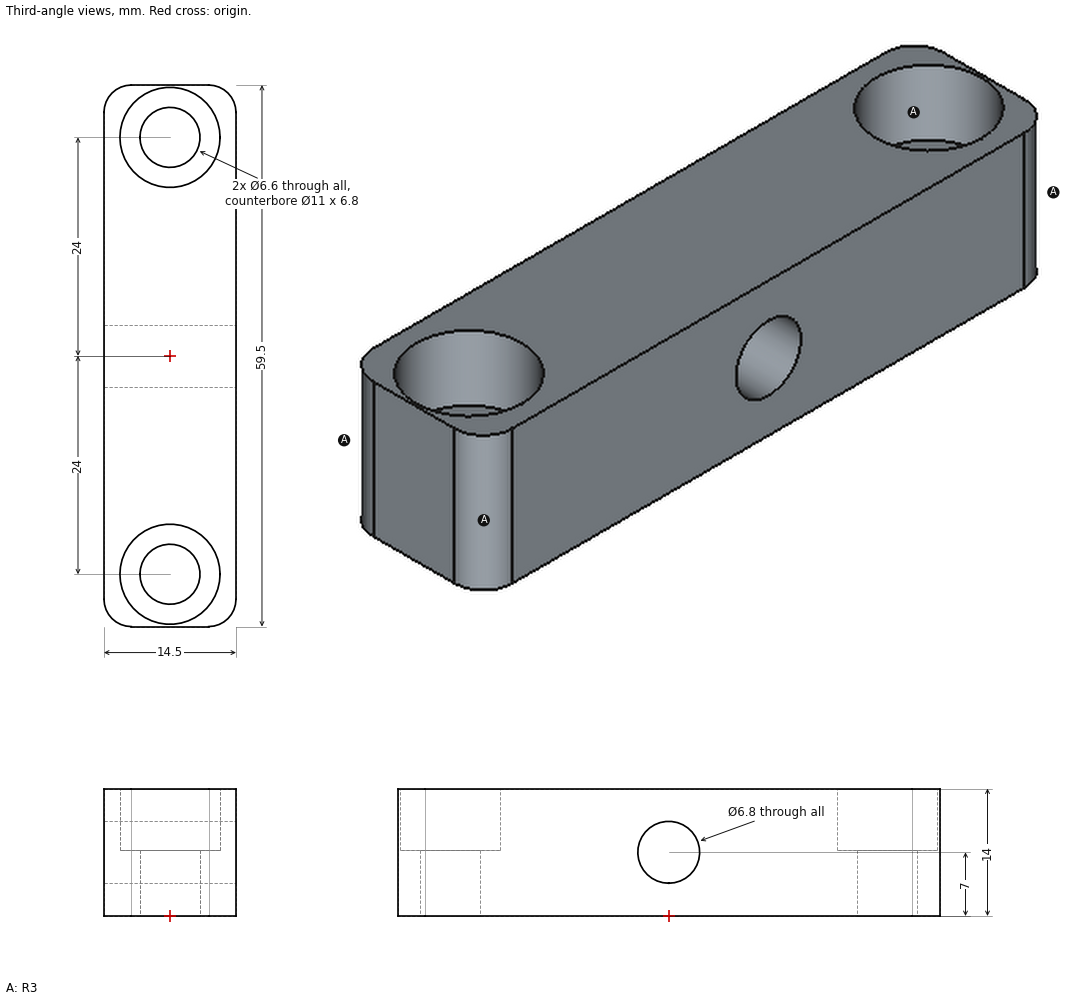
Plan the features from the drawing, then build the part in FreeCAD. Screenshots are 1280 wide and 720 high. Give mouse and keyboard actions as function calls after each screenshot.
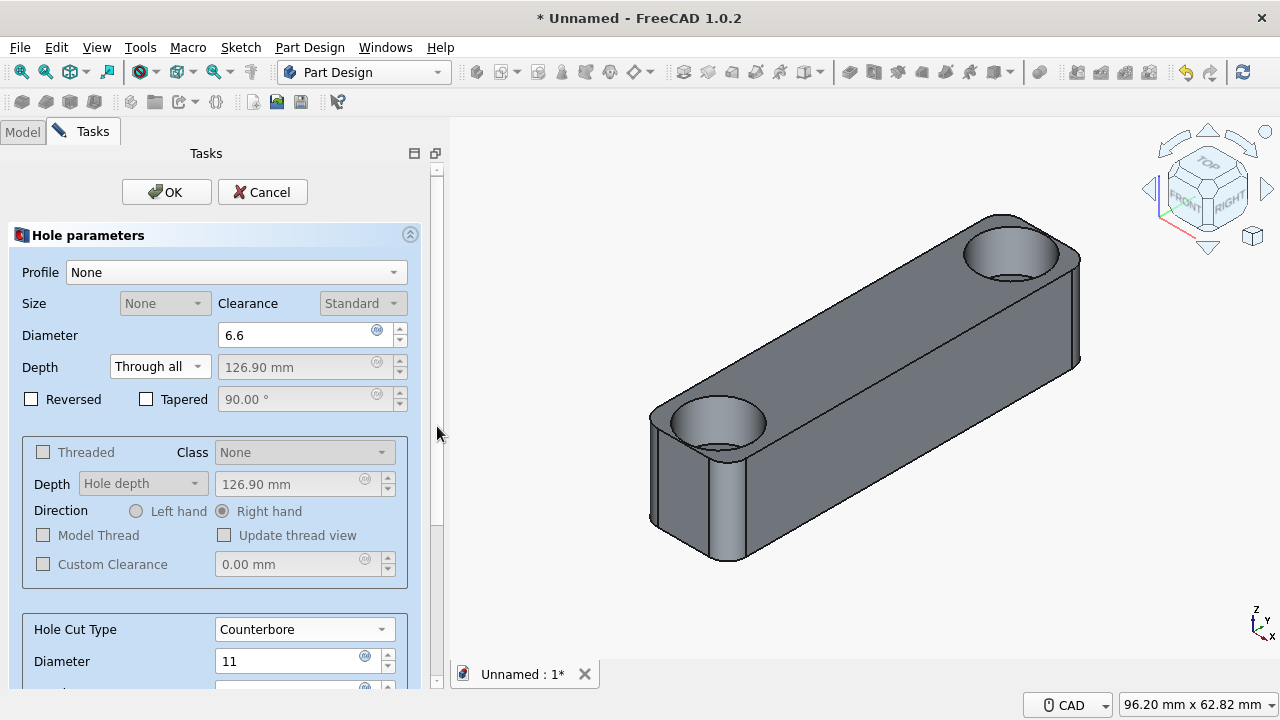
click(167, 192)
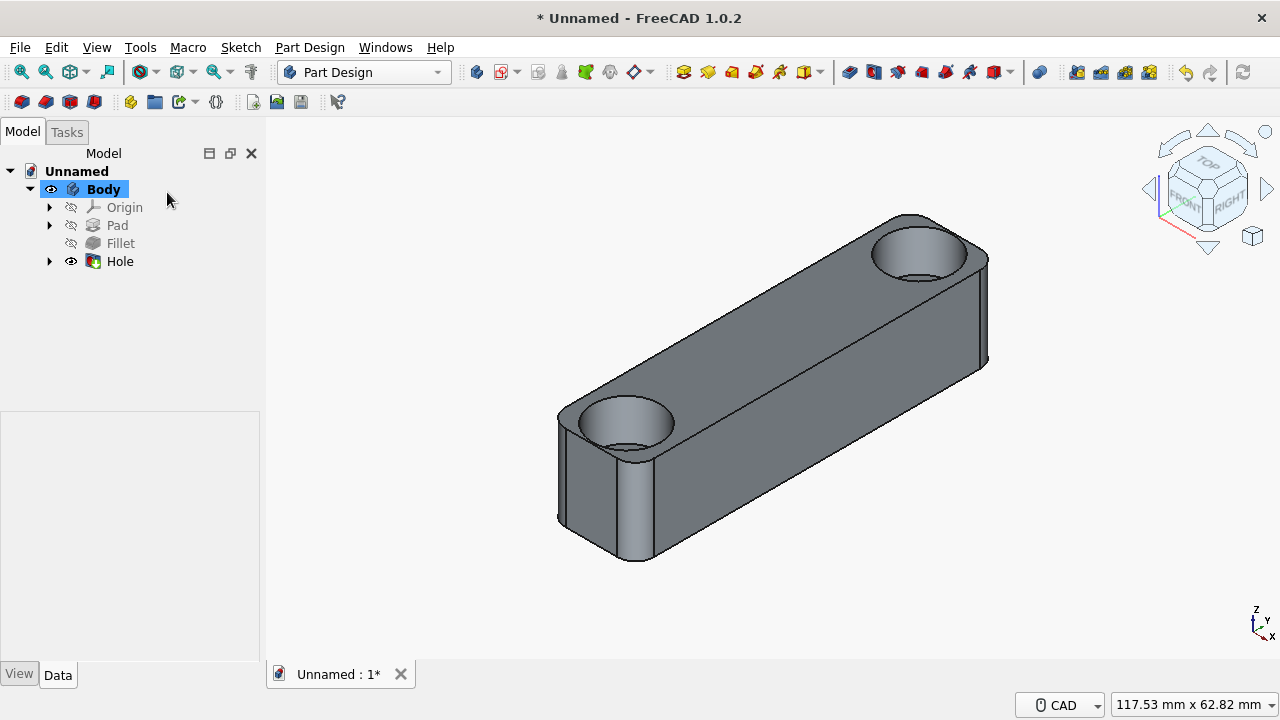
key(6)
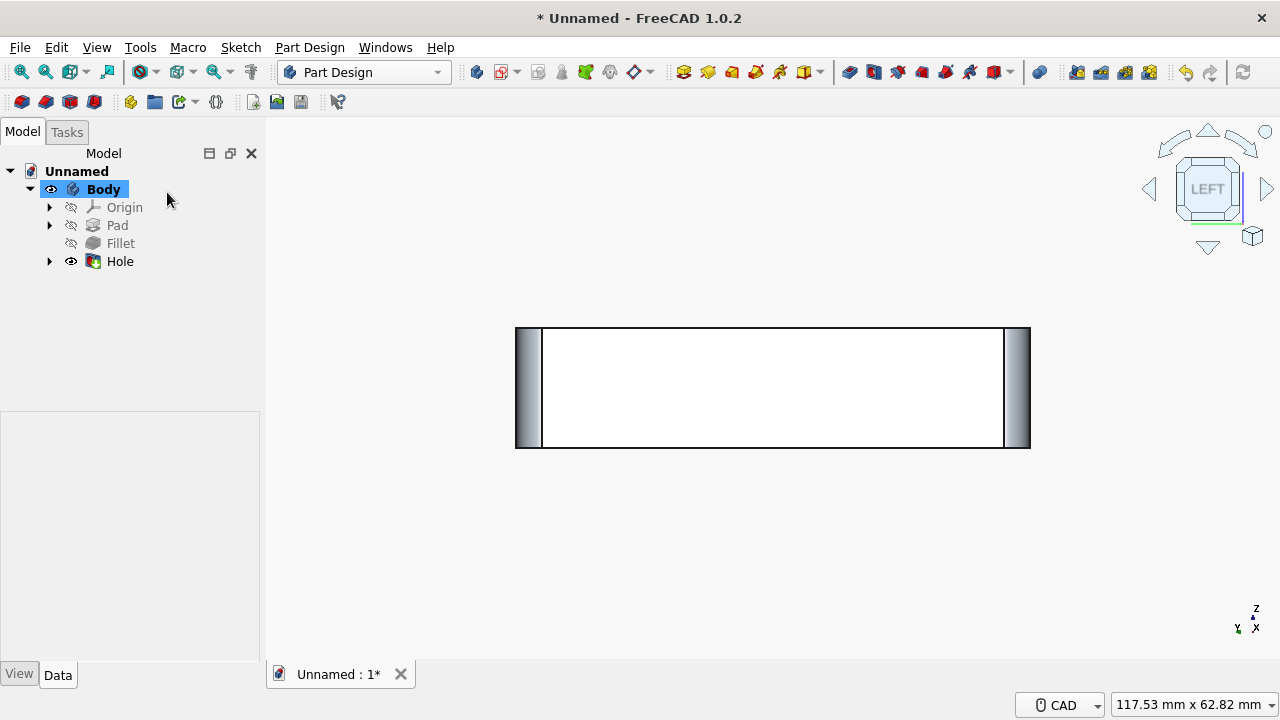
click(641, 387)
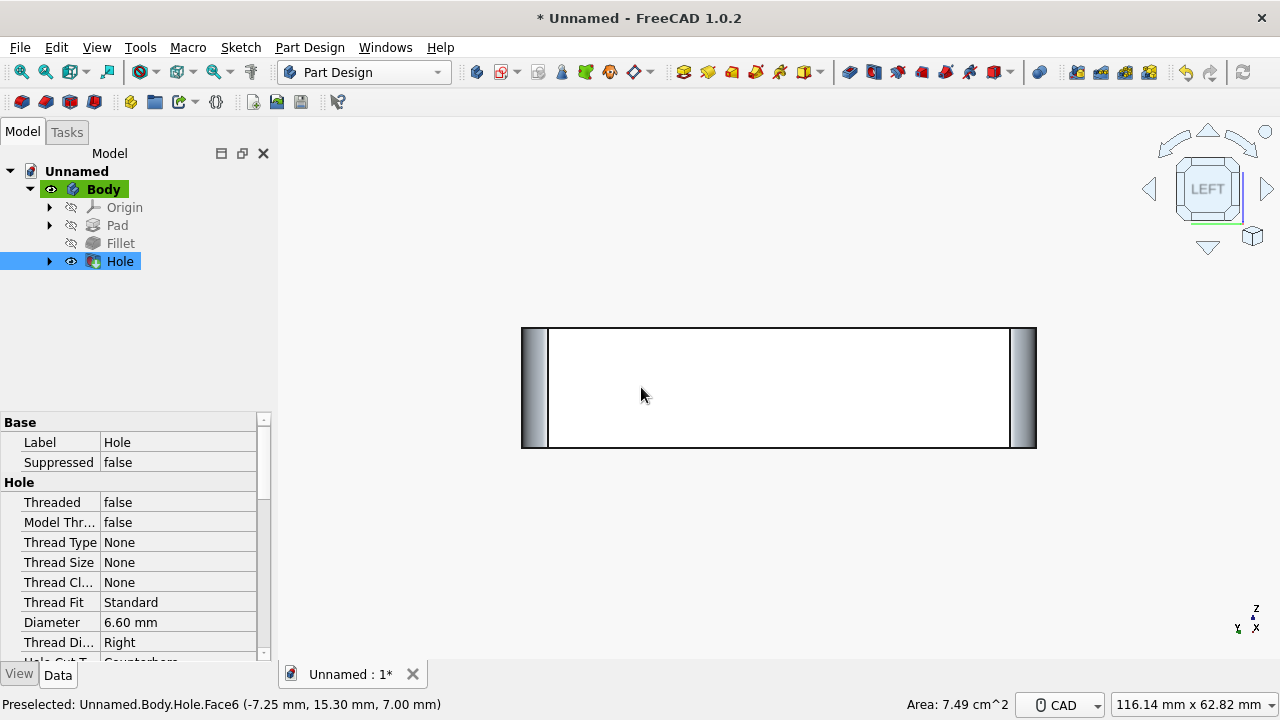
click(502, 72)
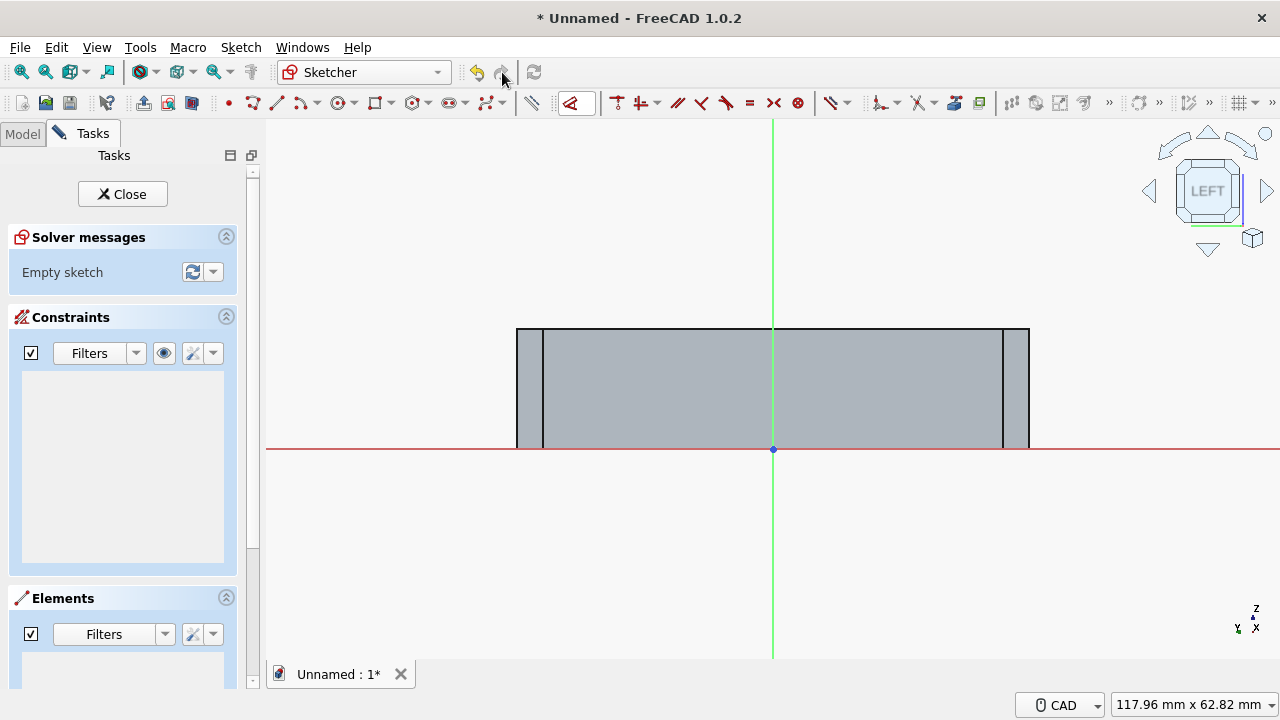
scroll(795, 410, up, 7)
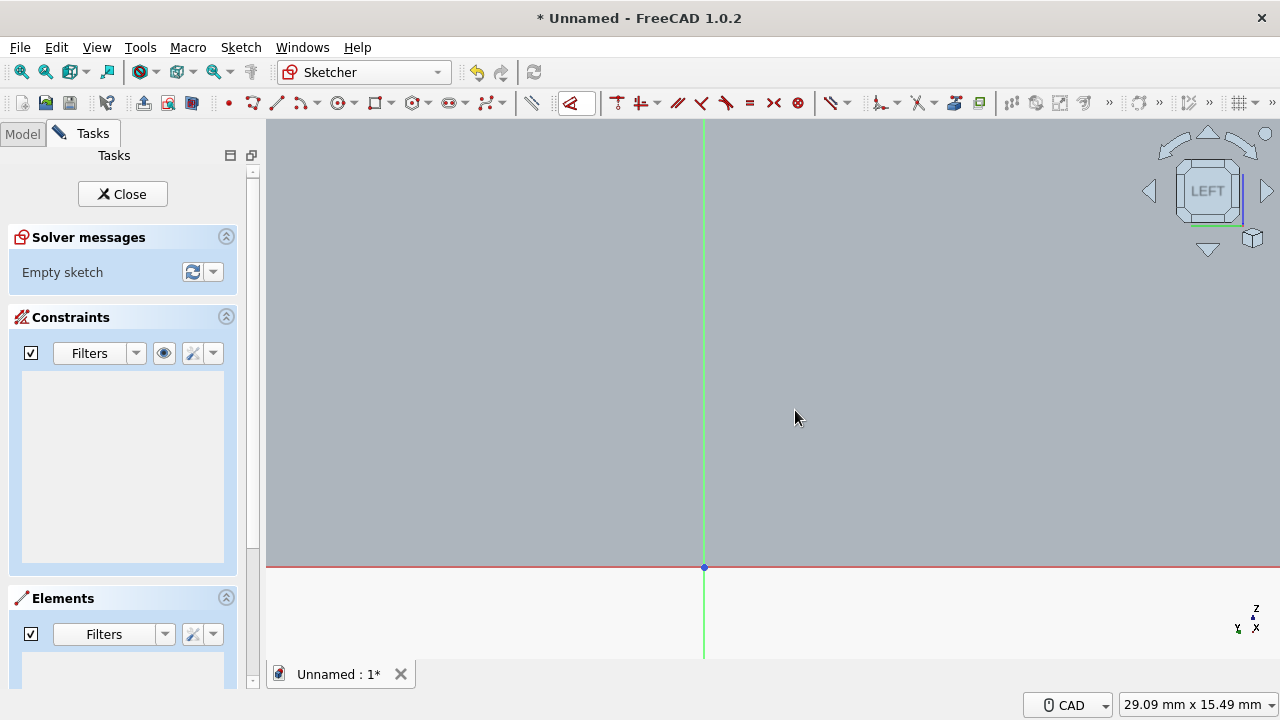
key(g)
key(c)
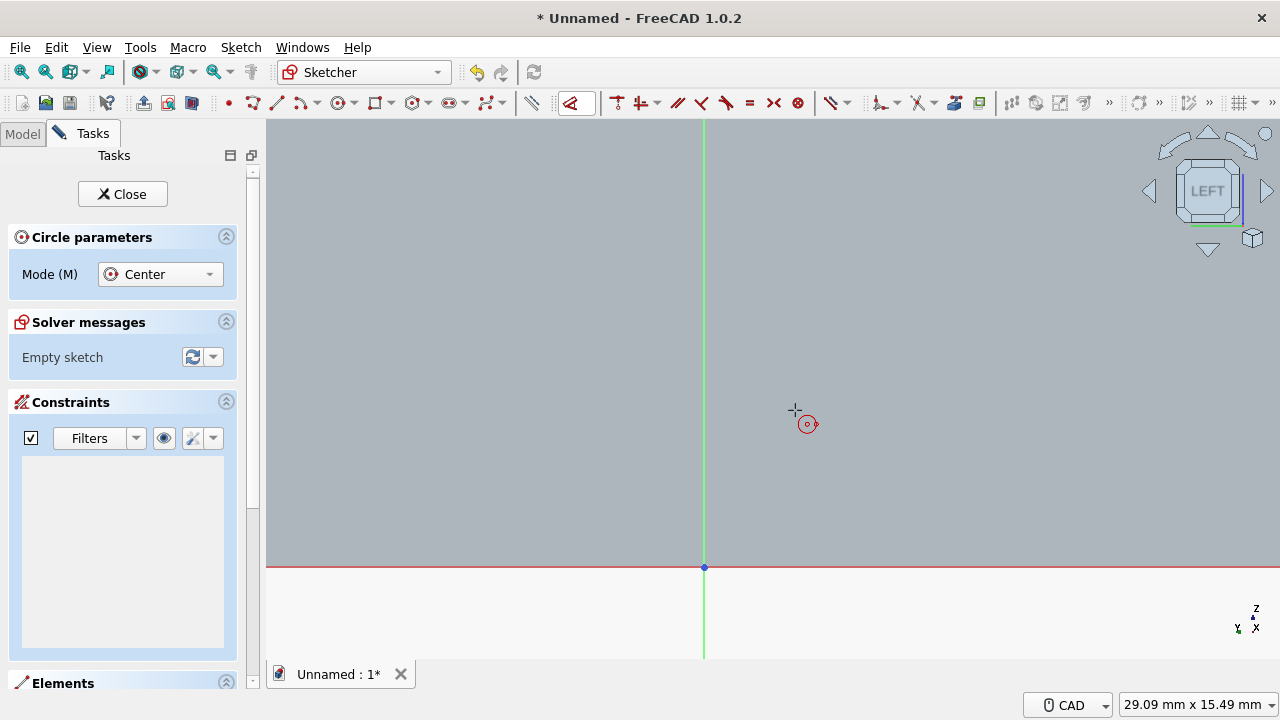
click(704, 323)
move(788, 239)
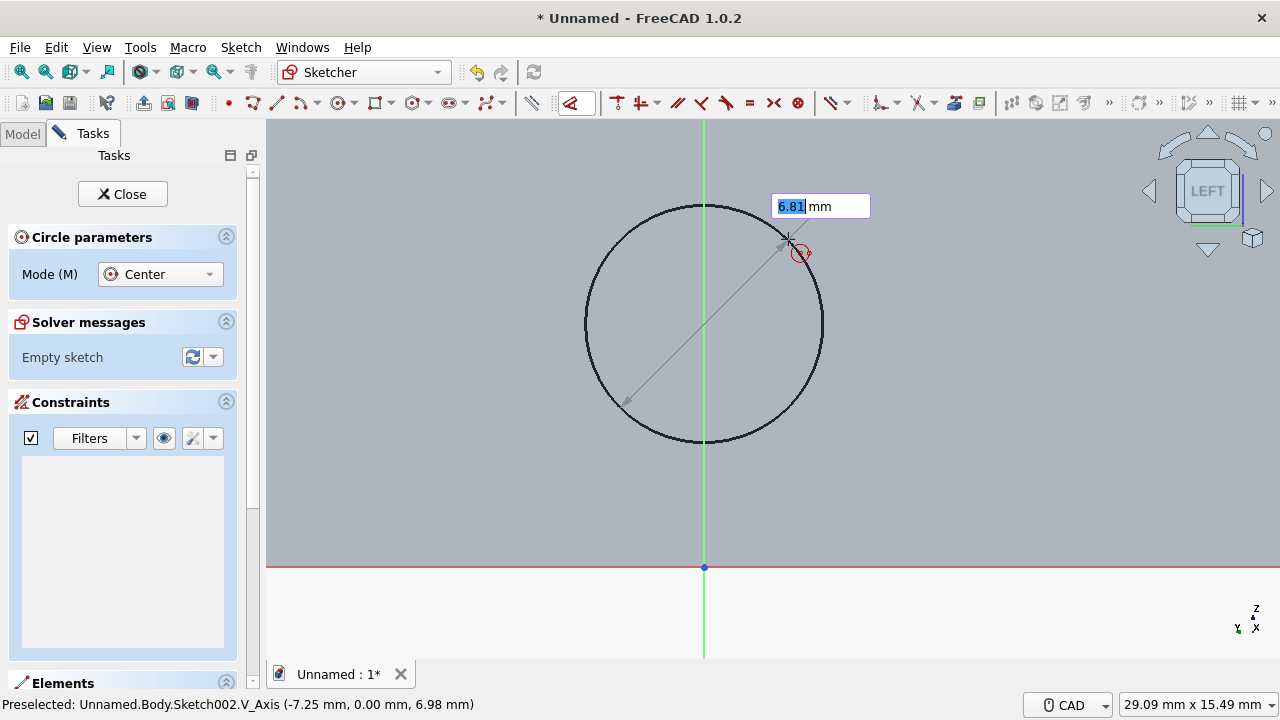
text(6.8)
key(Return)
key(Escape)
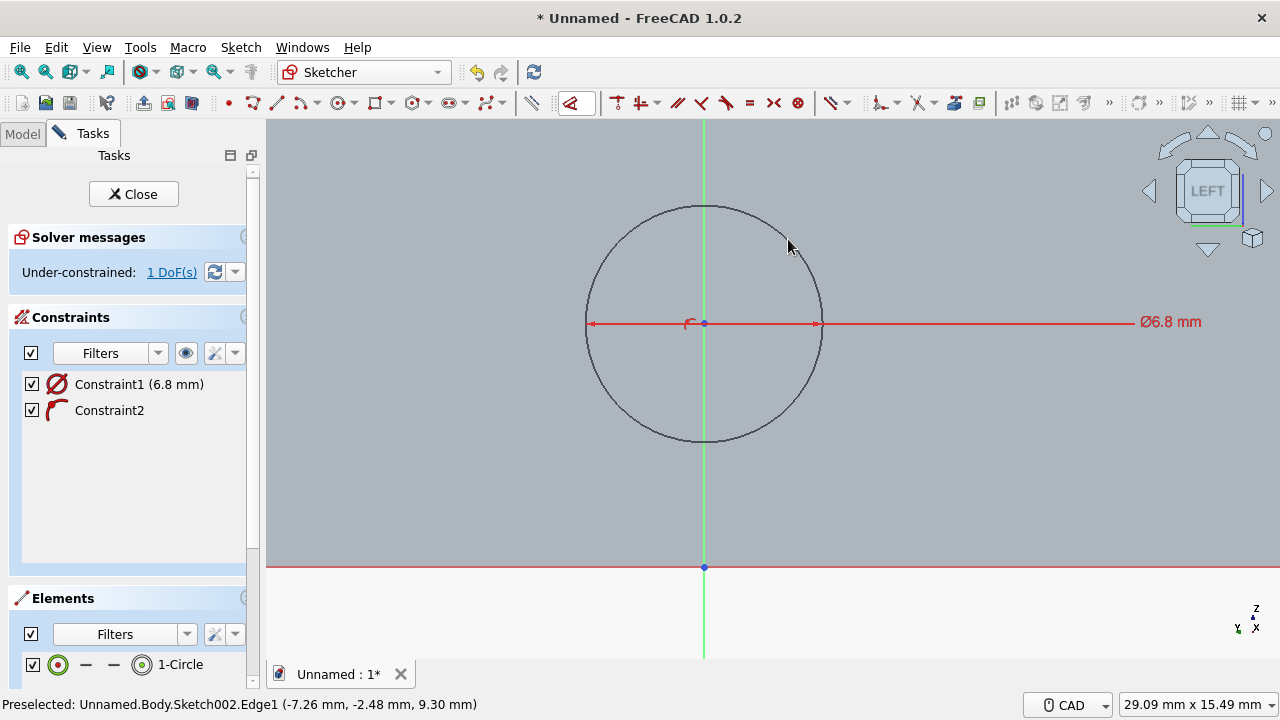
click(704, 324)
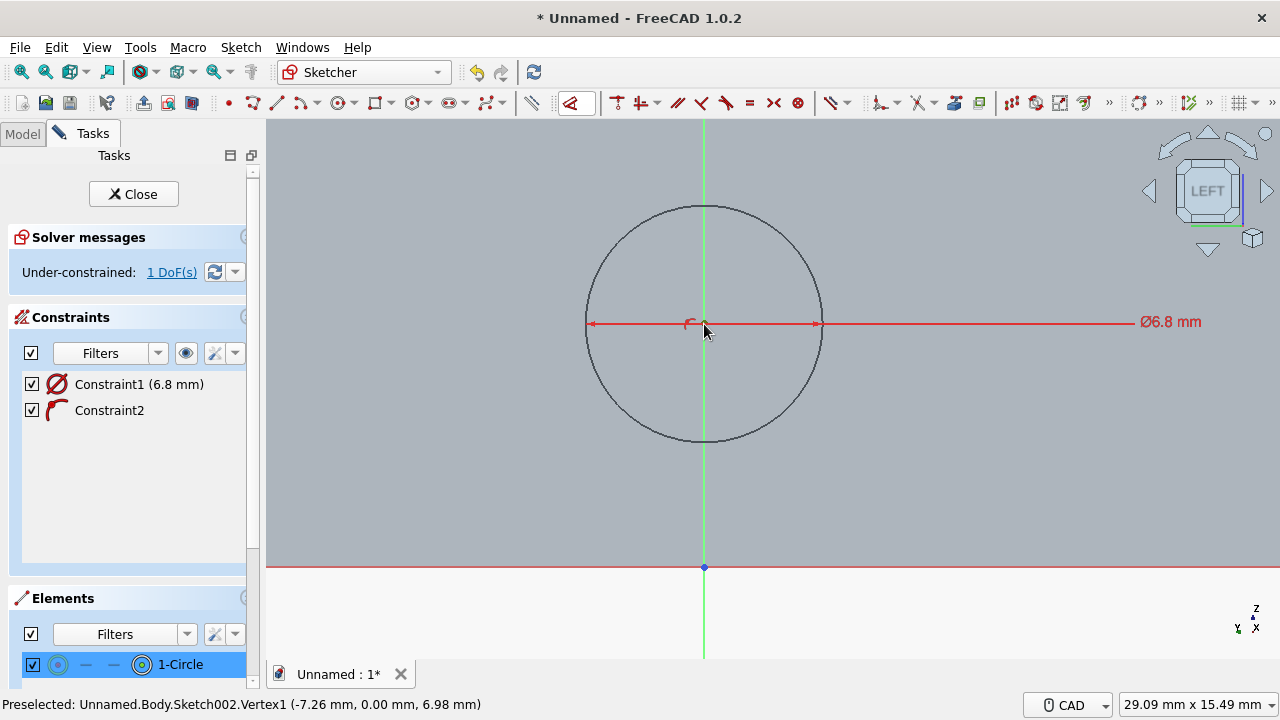
key(i)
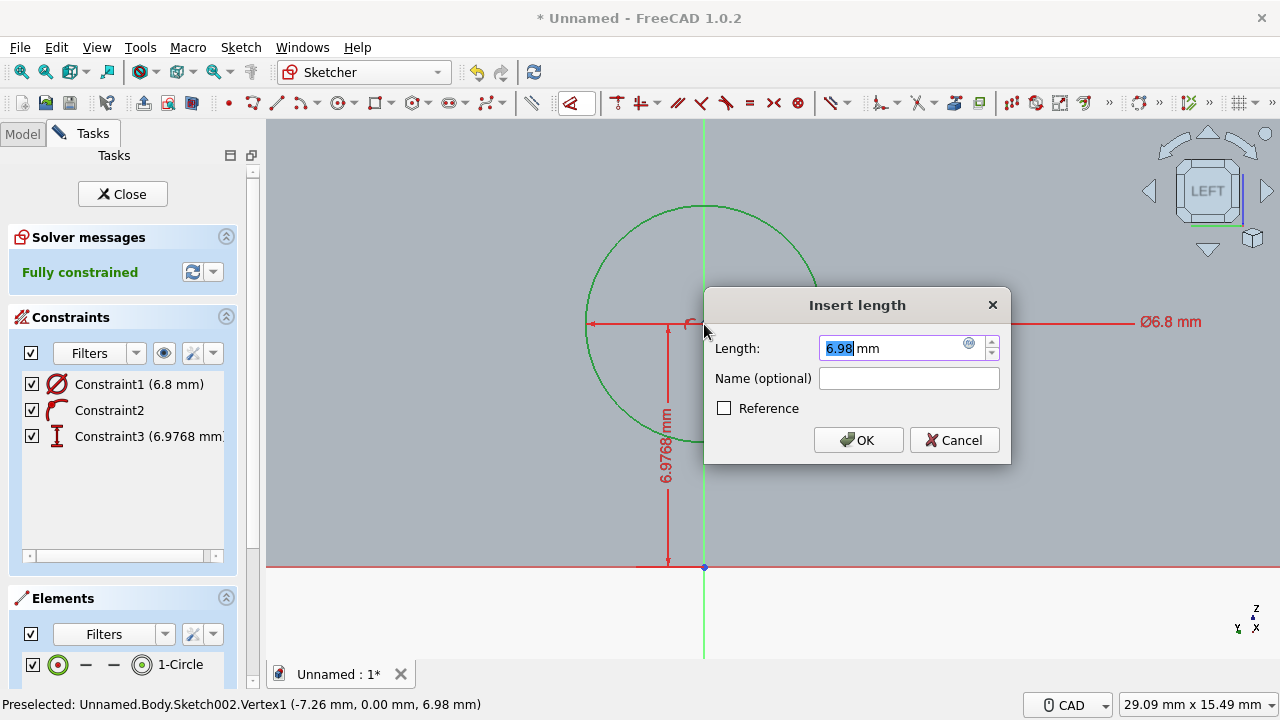
text(7)
key(Return)